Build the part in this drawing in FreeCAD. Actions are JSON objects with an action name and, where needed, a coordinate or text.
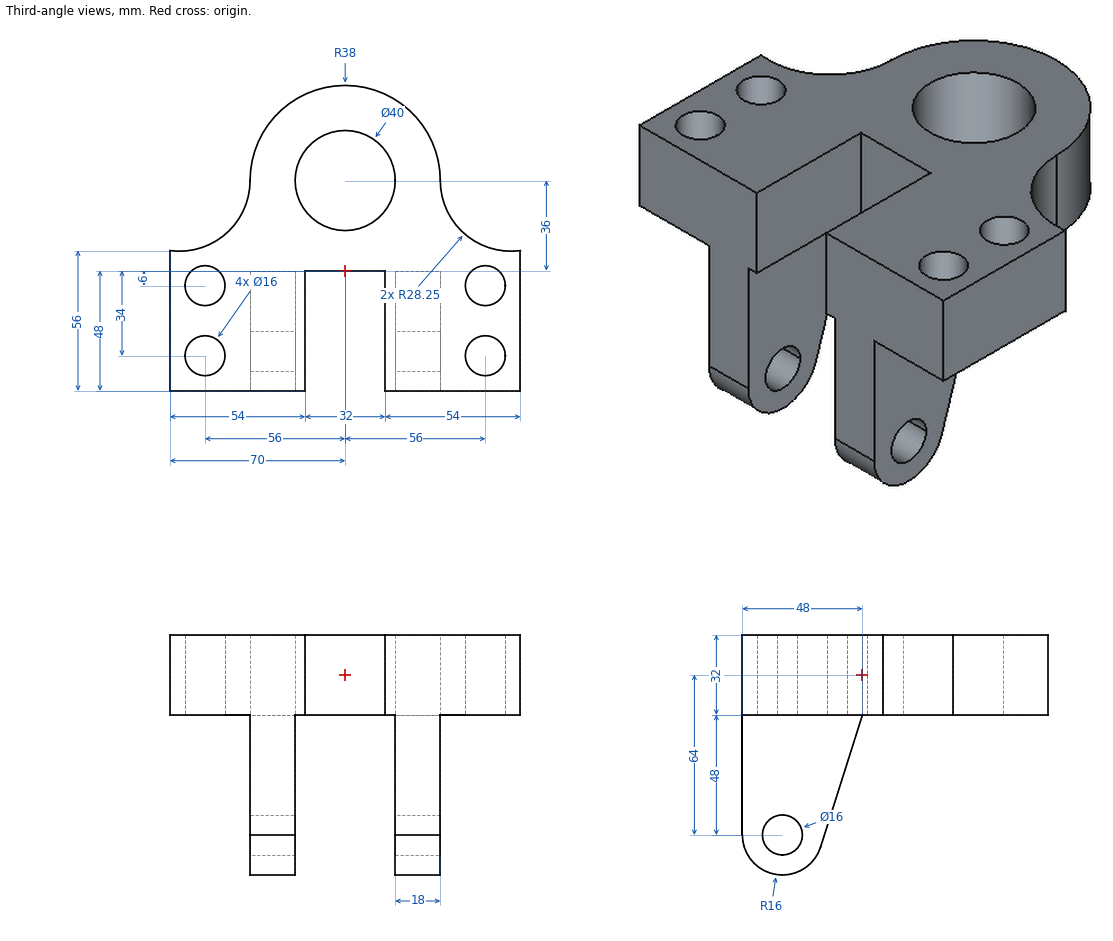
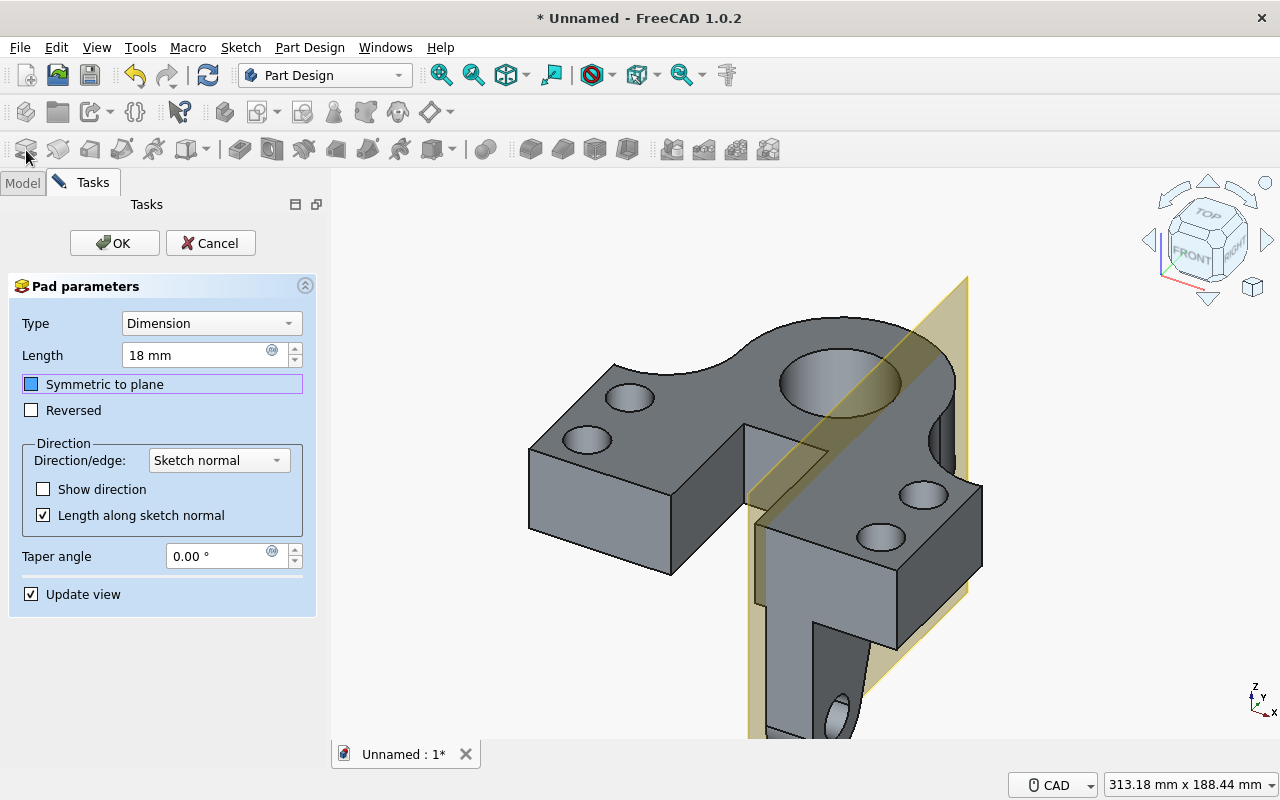
{"action": "left_click", "coordinate": [115, 243]}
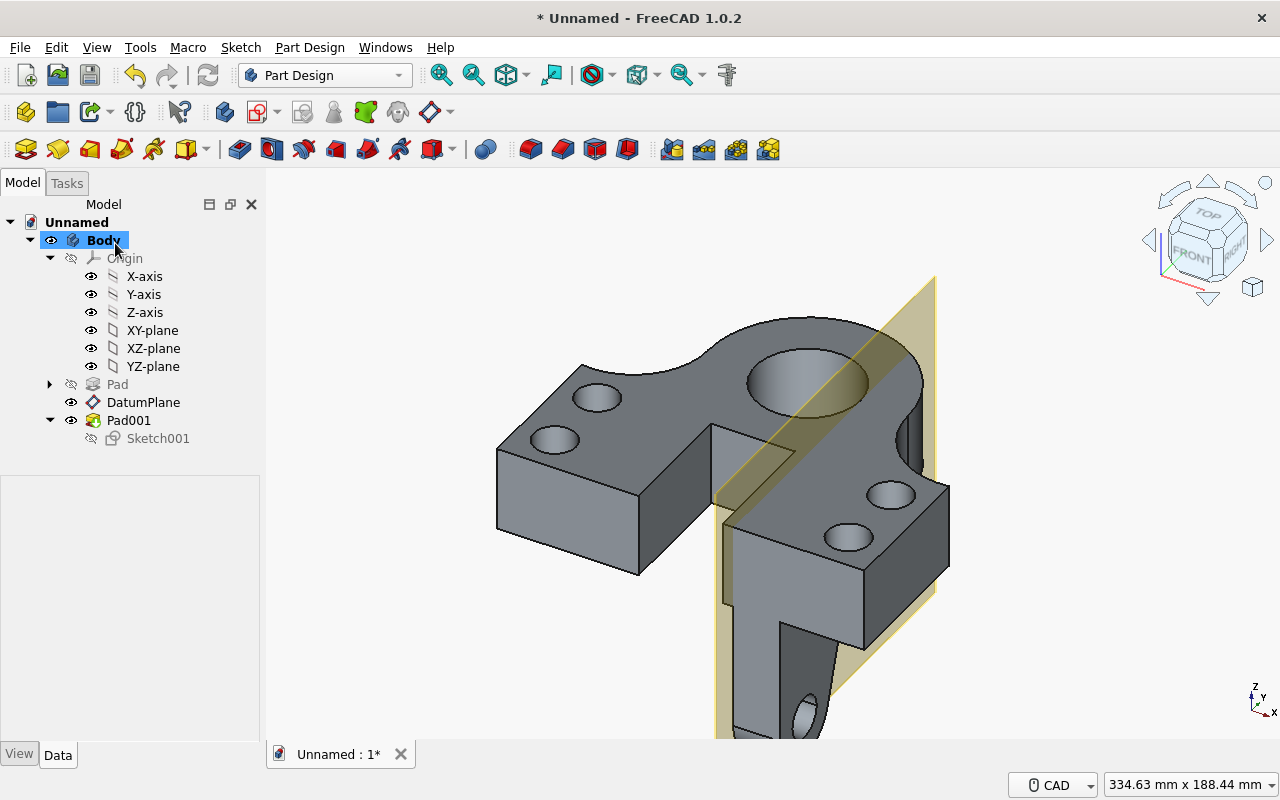
{"action": "left_click", "coordinate": [116, 402]}
{"action": "key", "text": "space"}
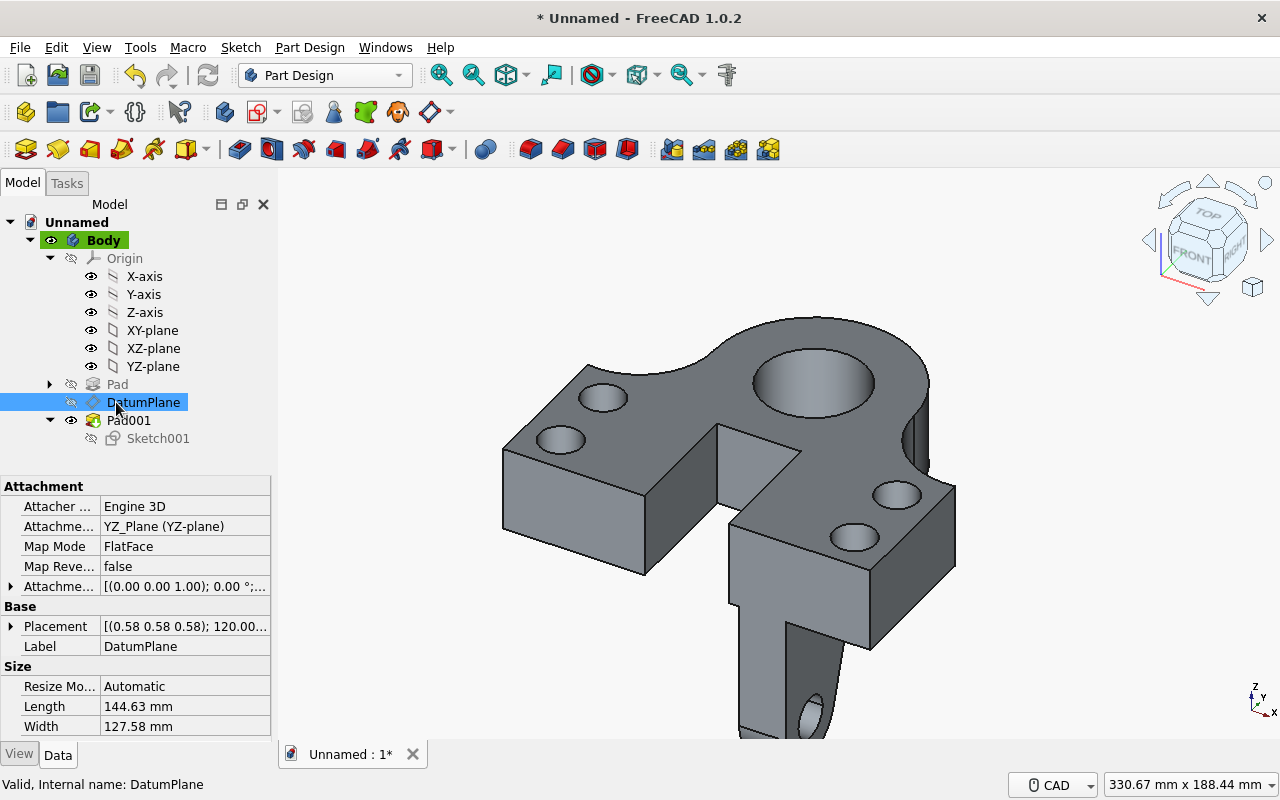
{"action": "left_click", "coordinate": [442, 76]}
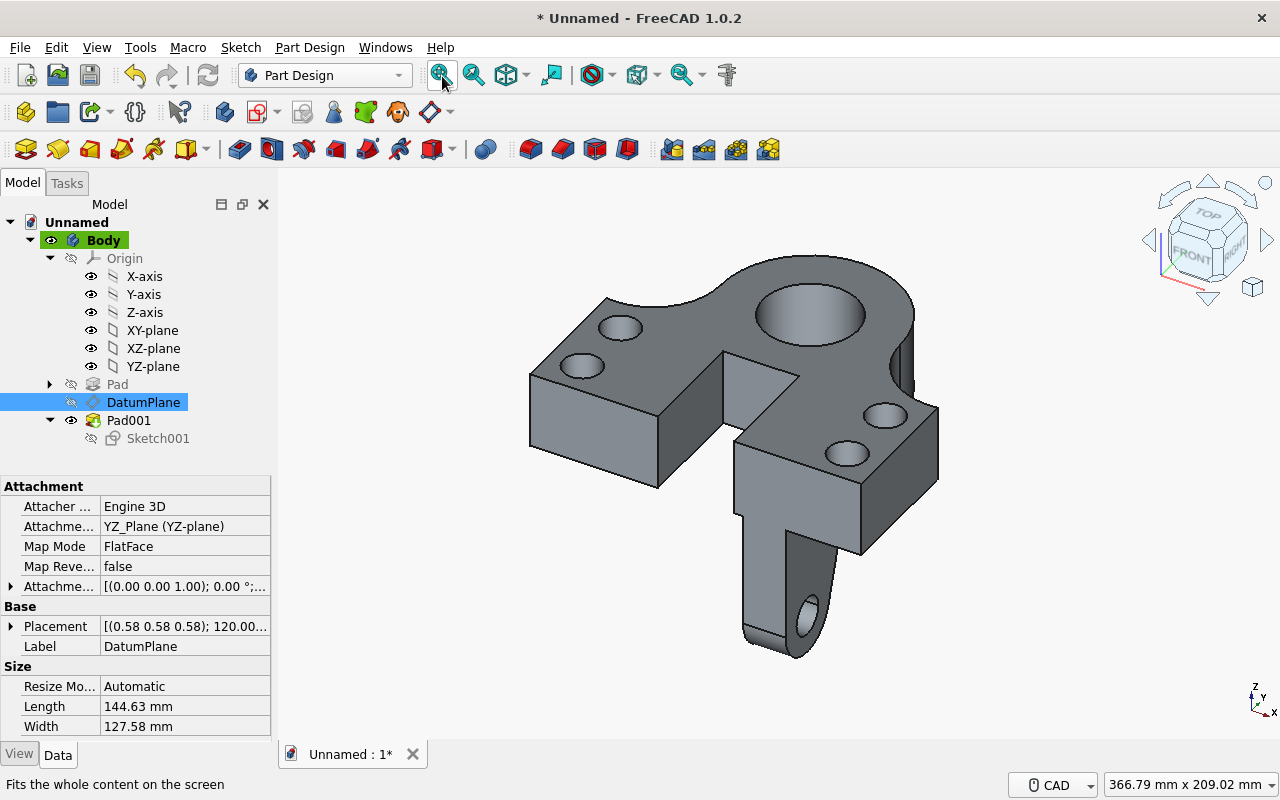
{"action": "left_click", "coordinate": [116, 420]}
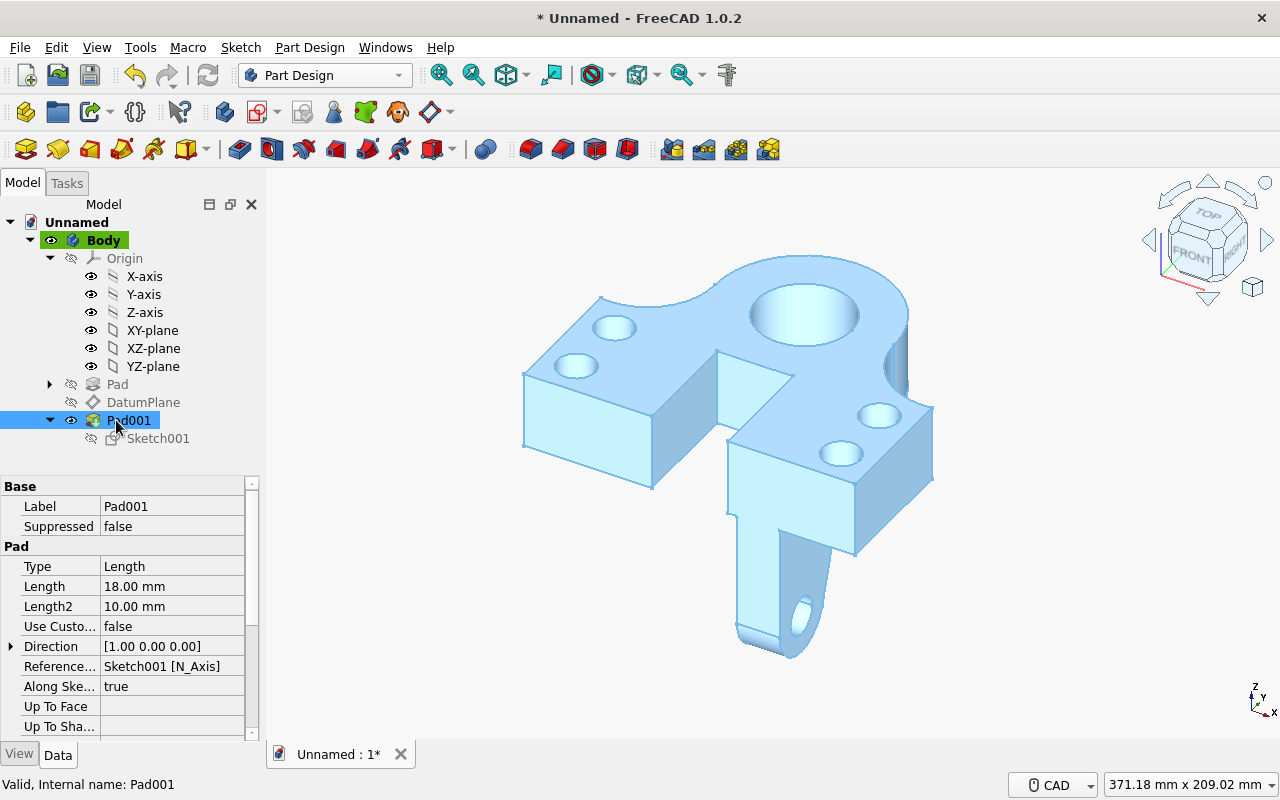
{"action": "left_click", "coordinate": [672, 150]}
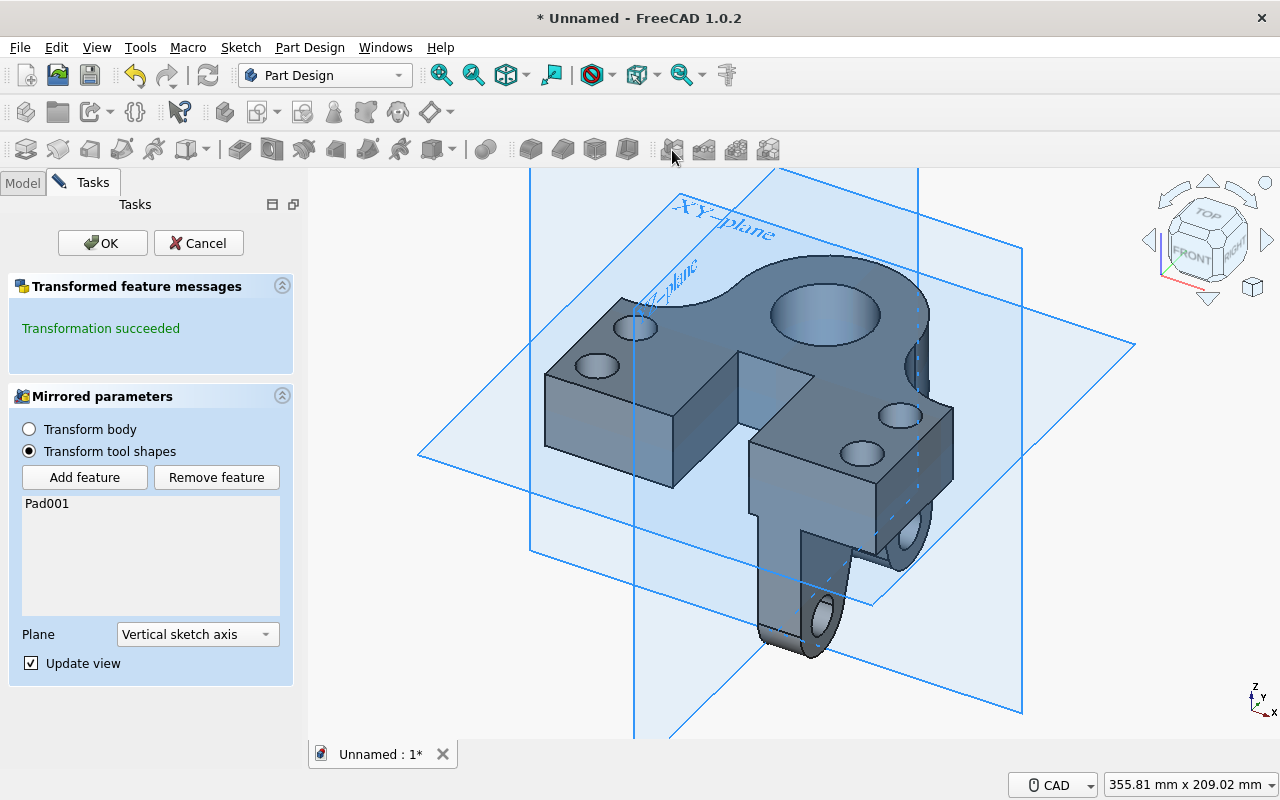
{"action": "left_click", "coordinate": [198, 634]}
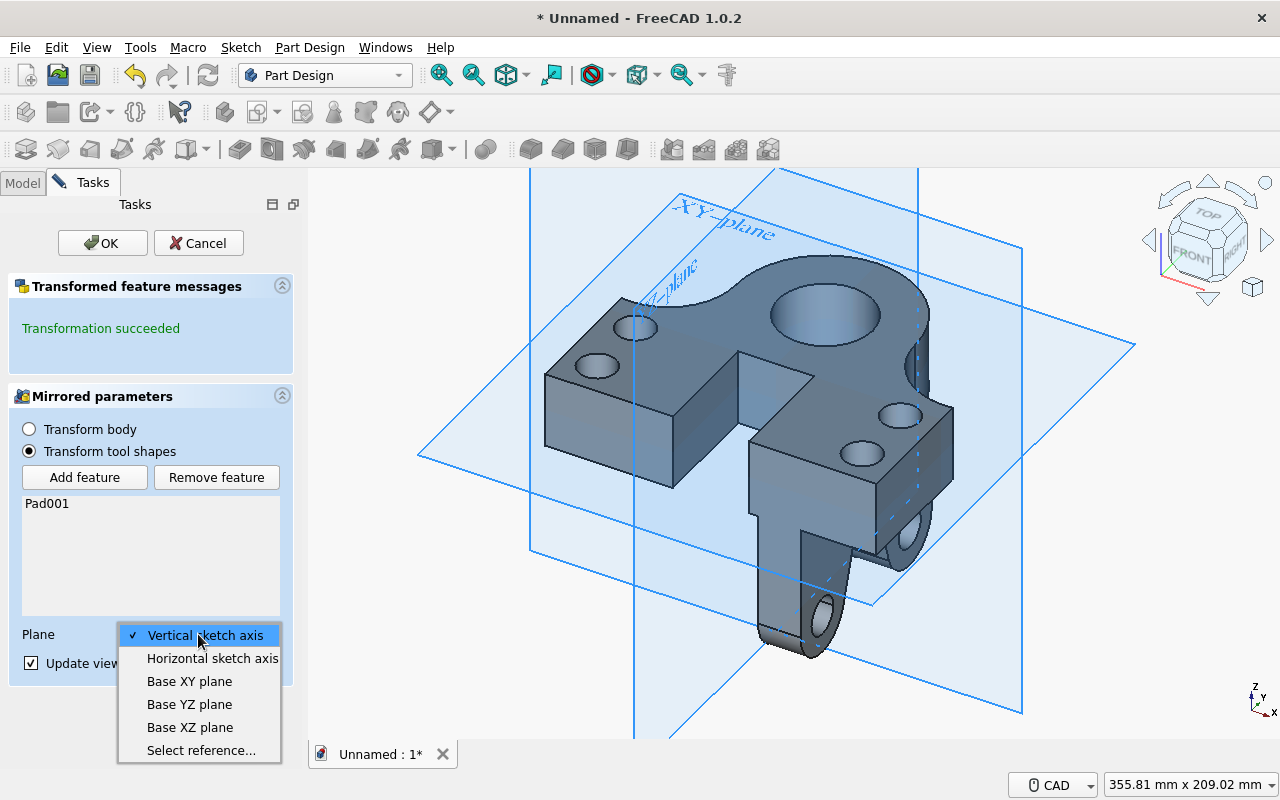
{"action": "left_click", "coordinate": [198, 704]}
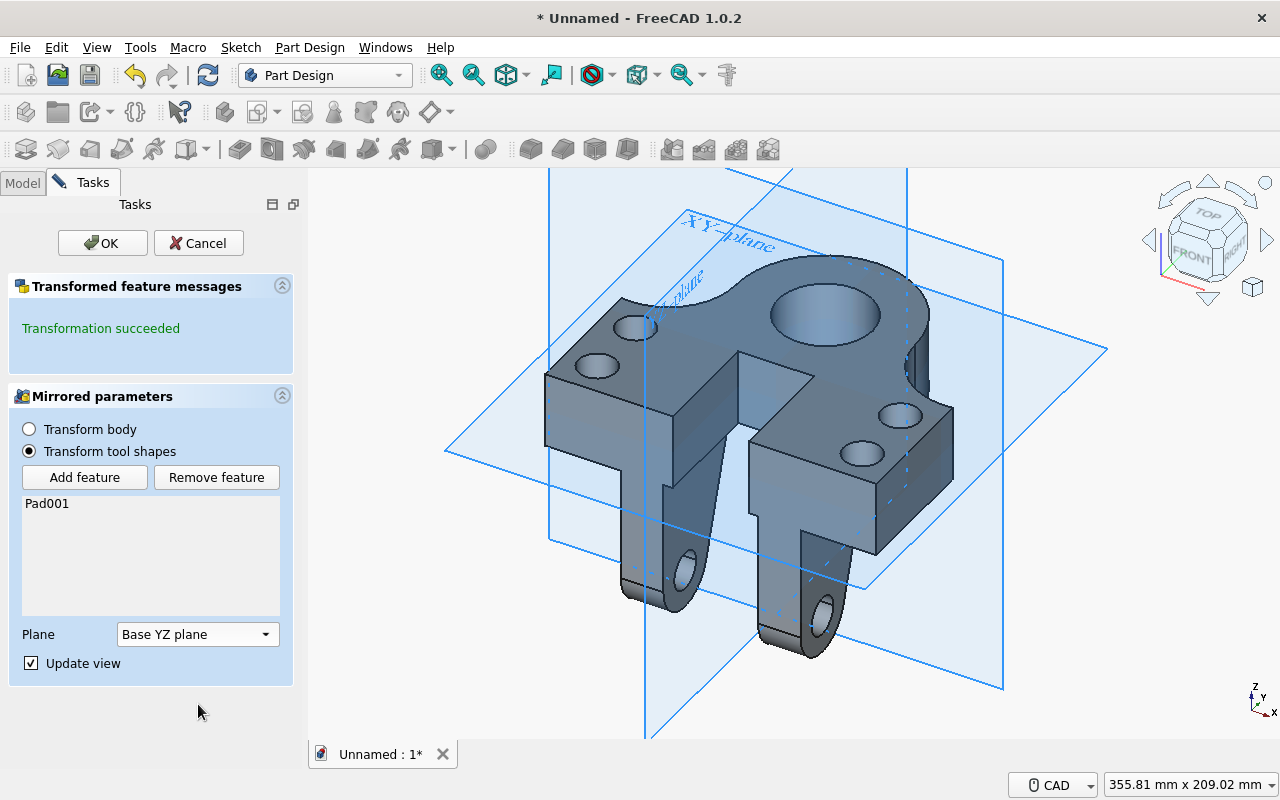
{"action": "left_click", "coordinate": [103, 243]}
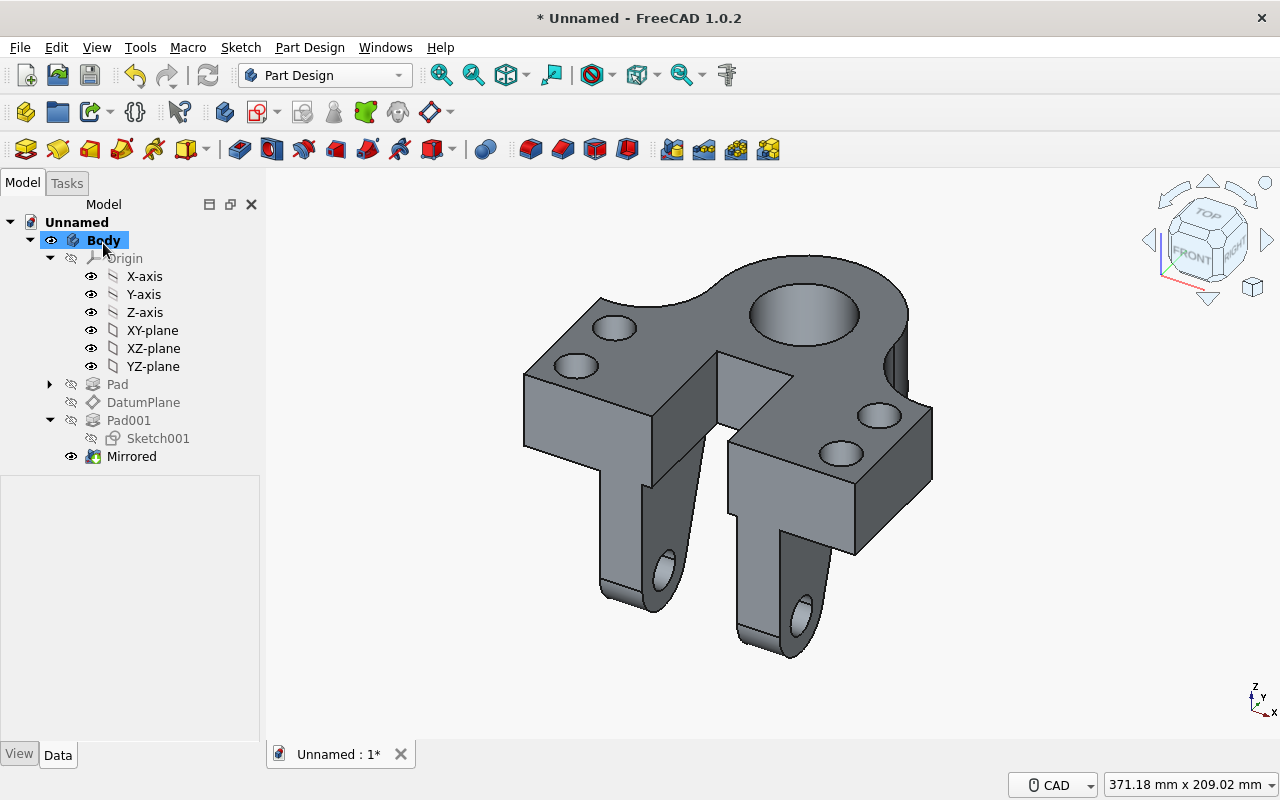
{"action": "key", "text": "0"}